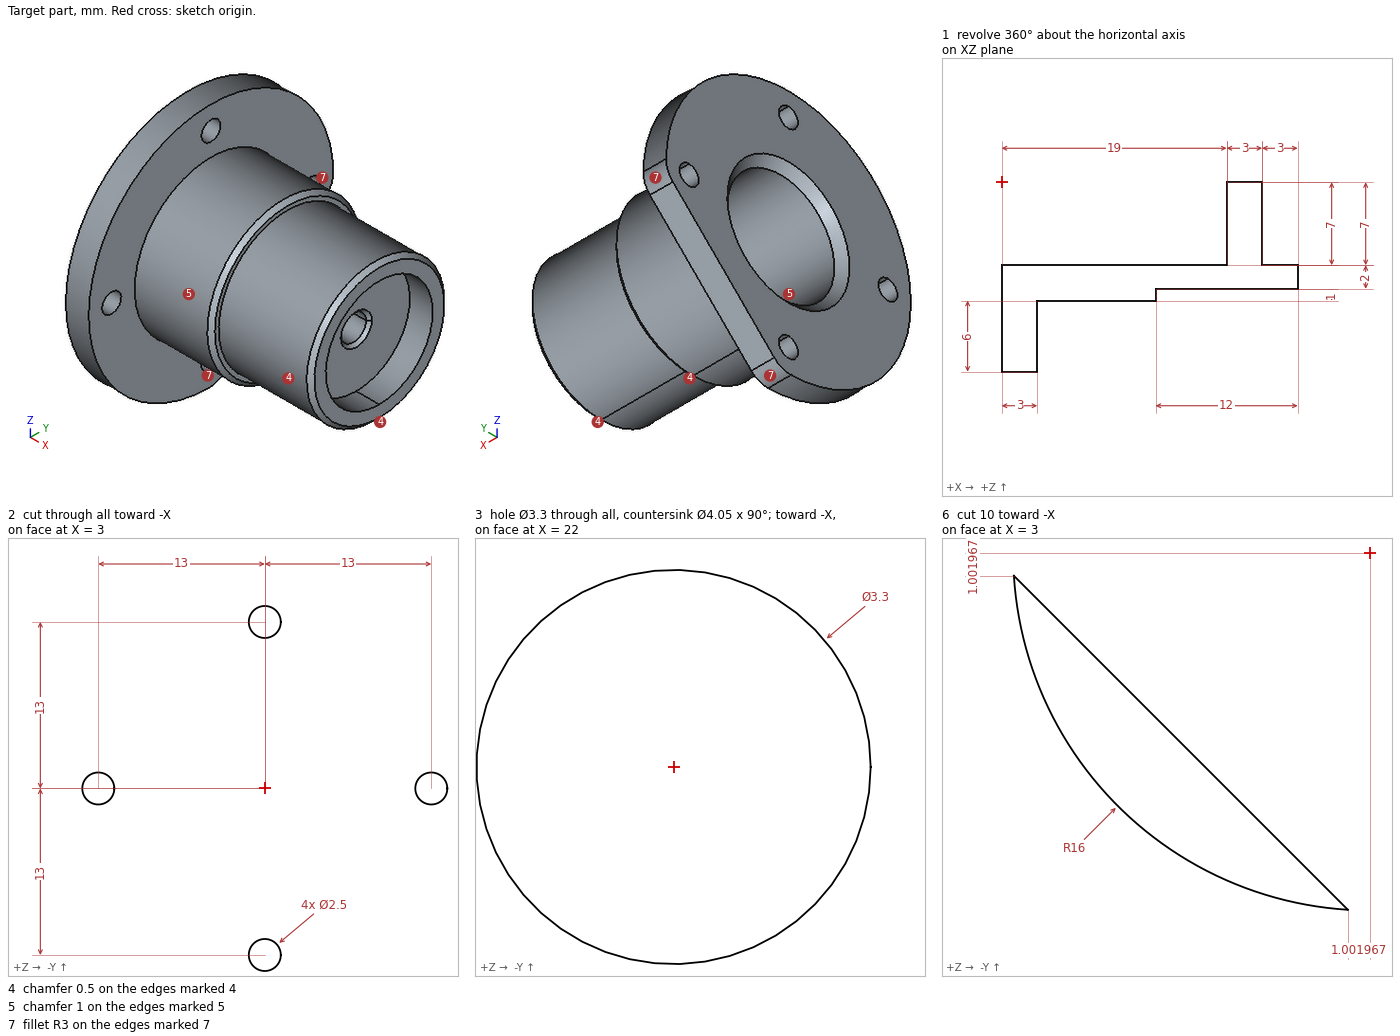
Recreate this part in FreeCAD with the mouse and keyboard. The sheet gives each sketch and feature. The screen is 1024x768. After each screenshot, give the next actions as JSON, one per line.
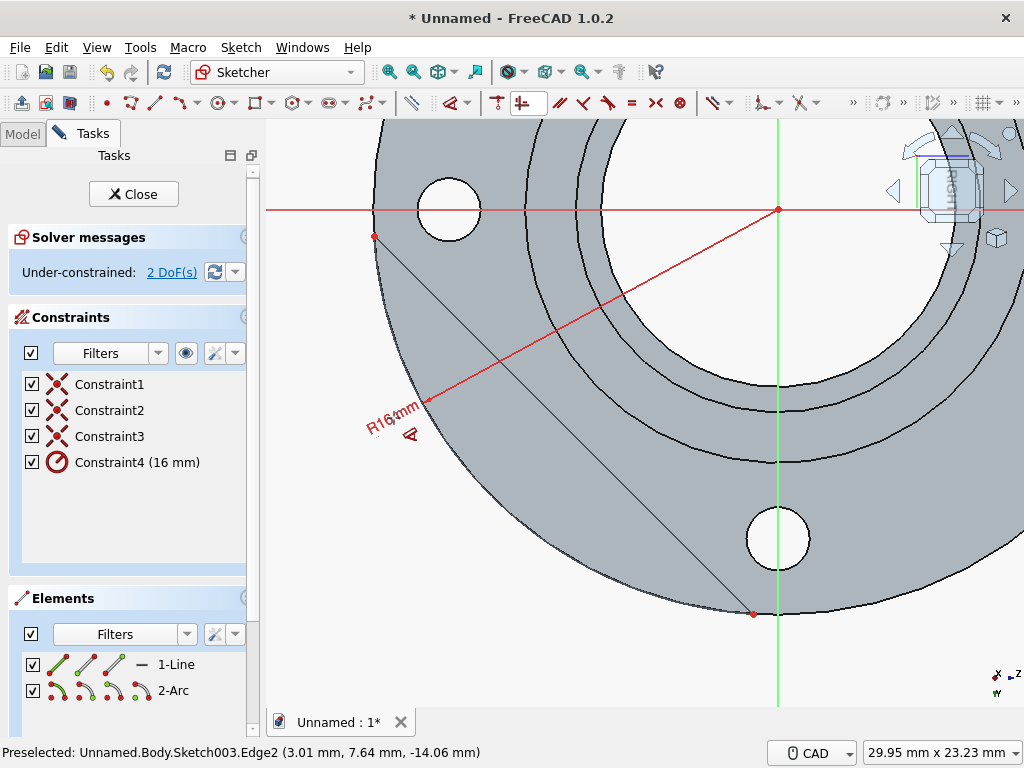
{"action": "scroll", "coordinate": [753, 614], "scroll_direction": "up", "scroll_amount": 3}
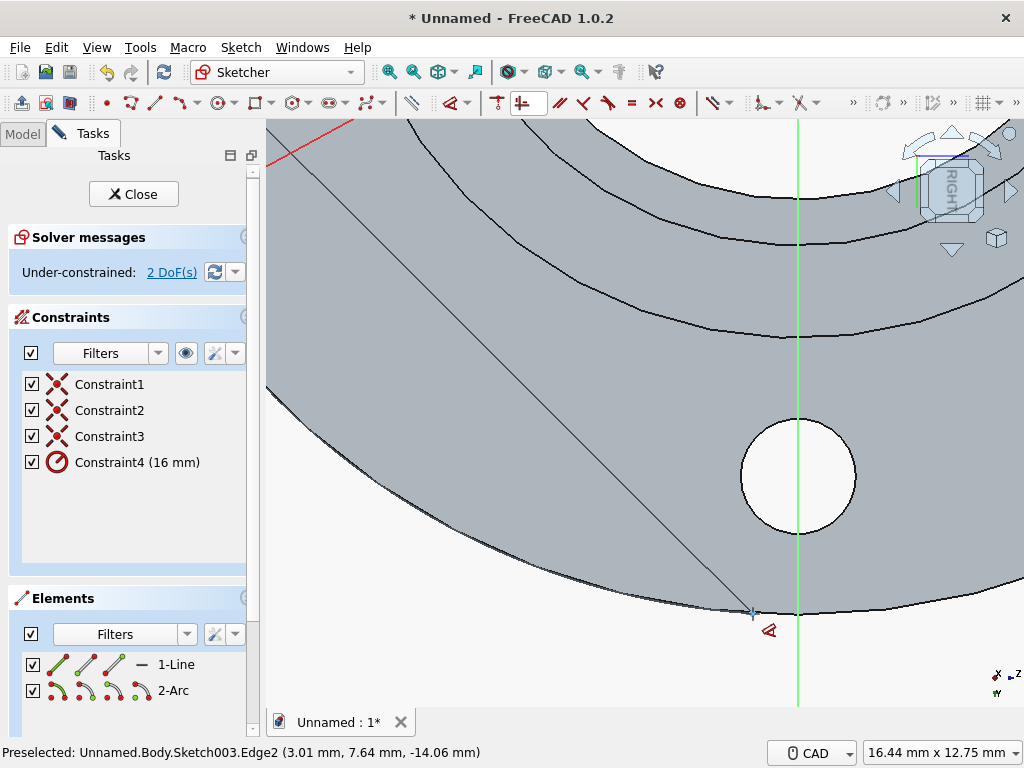
{"action": "left_click", "coordinate": [752, 613]}
{"action": "left_click", "coordinate": [775, 647]}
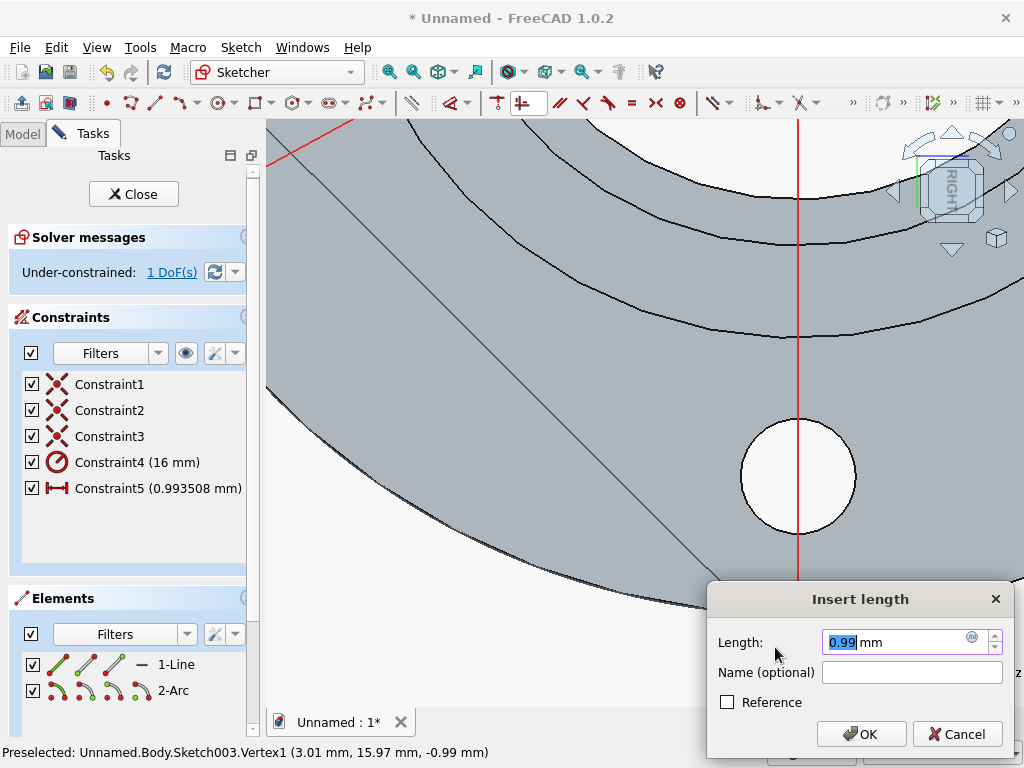
{"action": "type", "text": "1.001967"}
{"action": "key", "text": "Return"}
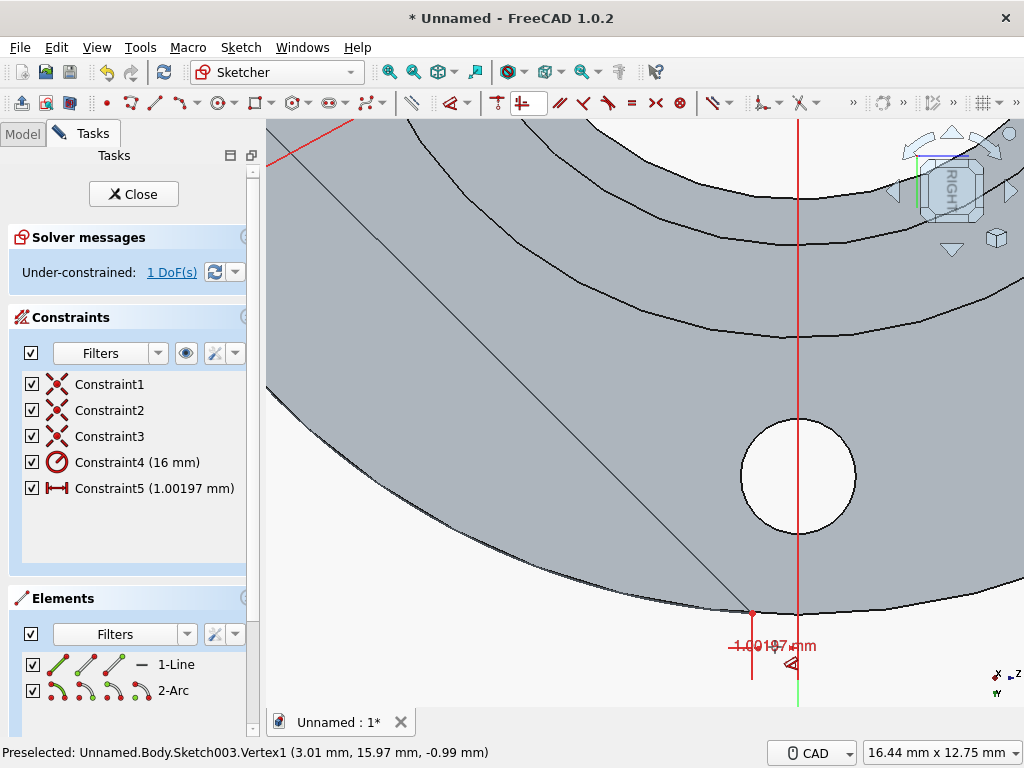
{"action": "scroll", "coordinate": [755, 617], "scroll_direction": "down", "scroll_amount": 3}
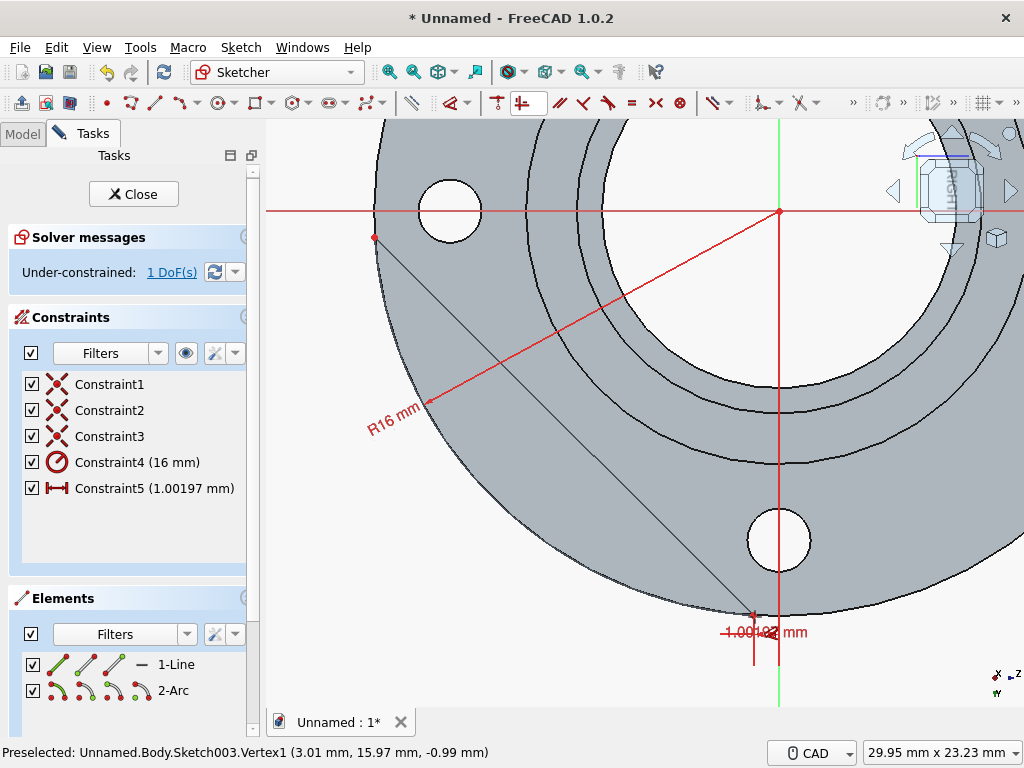
{"action": "scroll", "coordinate": [375, 237], "scroll_direction": "up", "scroll_amount": 3}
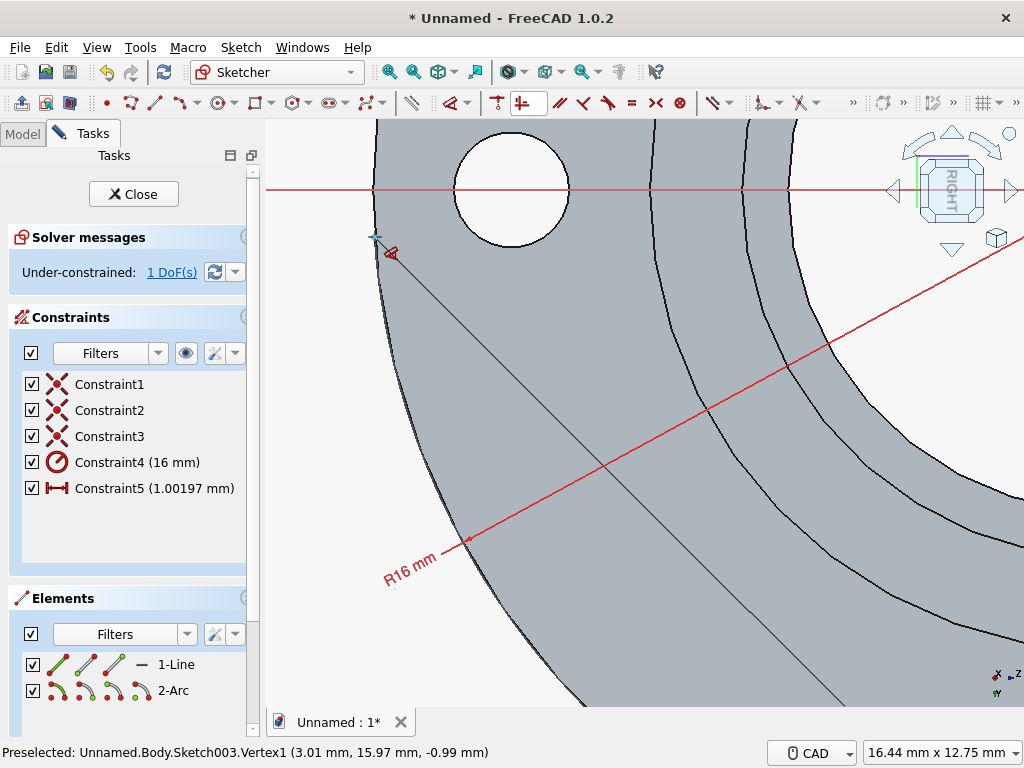
{"action": "left_click", "coordinate": [375, 237]}
{"action": "left_click", "coordinate": [341, 214]}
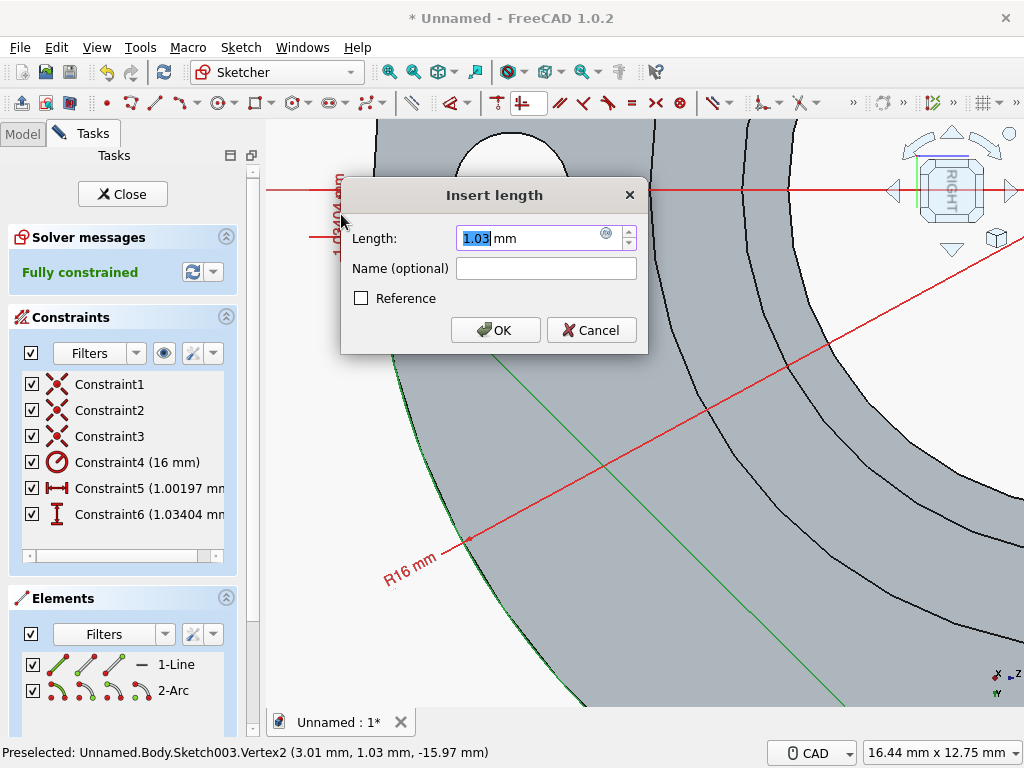
{"action": "type", "text": "1.001967"}
{"action": "key", "text": "Return"}
{"action": "key", "text": "Escape"}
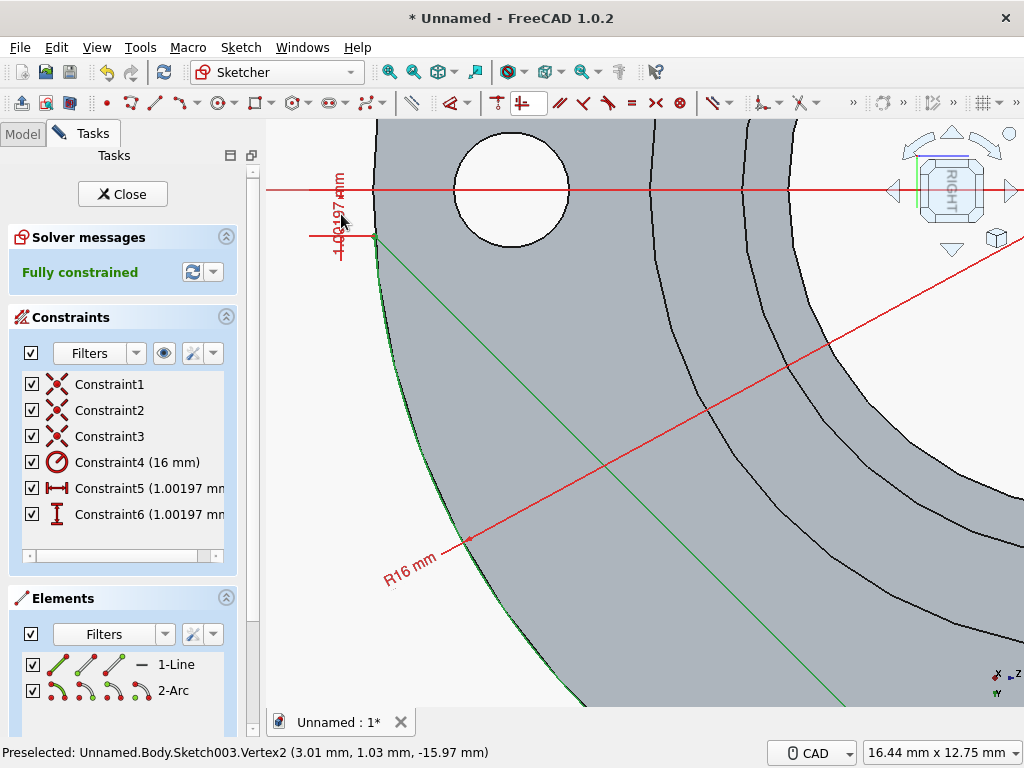
{"action": "left_click", "coordinate": [123, 194]}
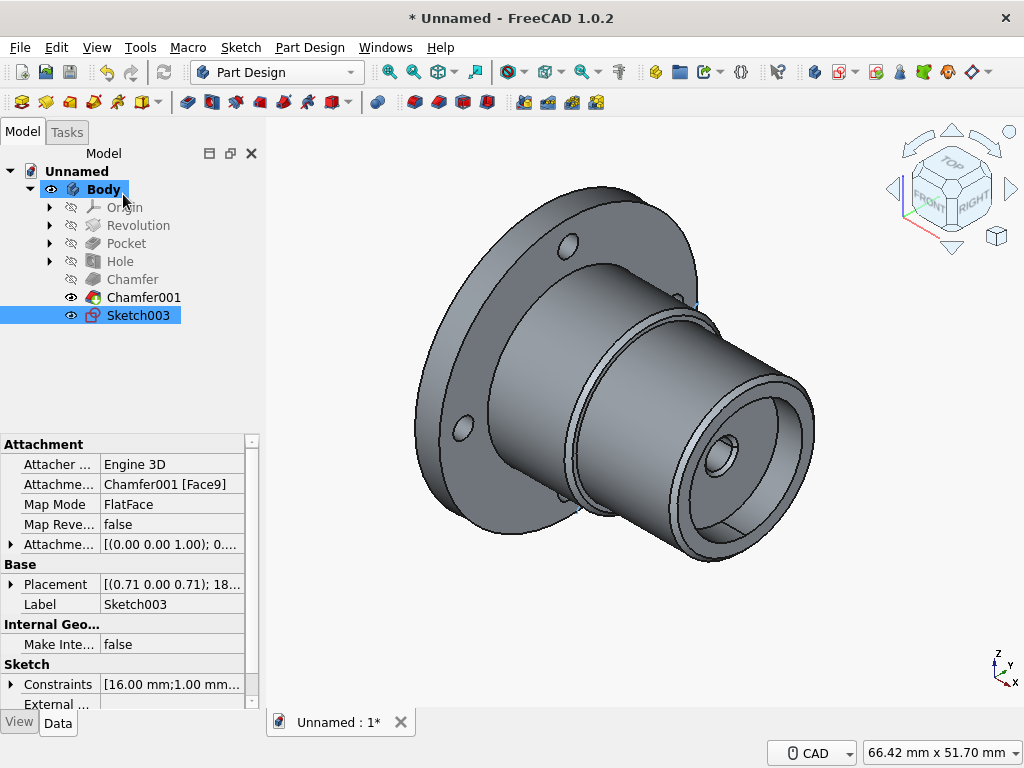
{"action": "left_click", "coordinate": [188, 102]}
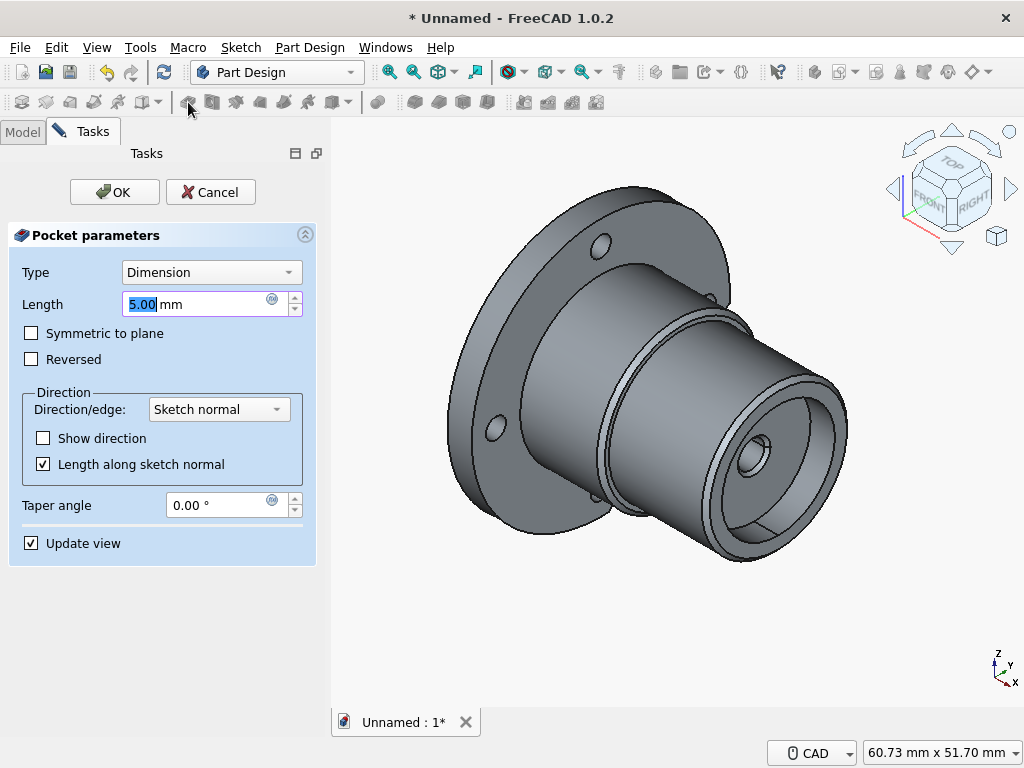
{"action": "type", "text": "10"}
{"action": "key", "text": "Tab"}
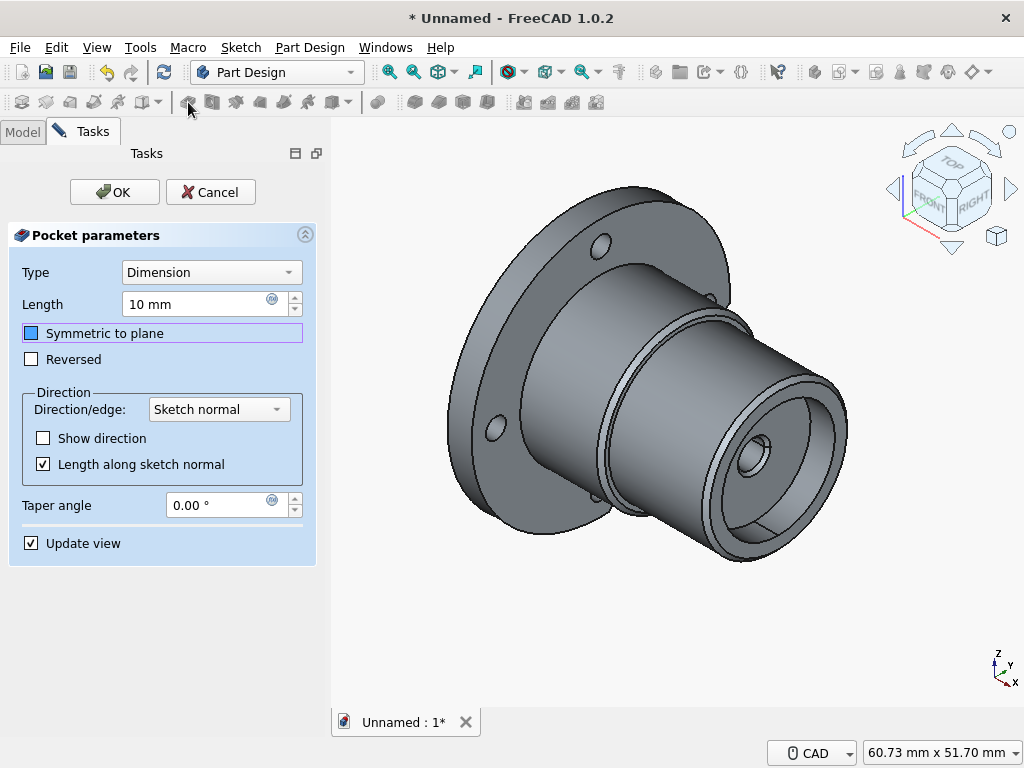
{"action": "left_click", "coordinate": [115, 192]}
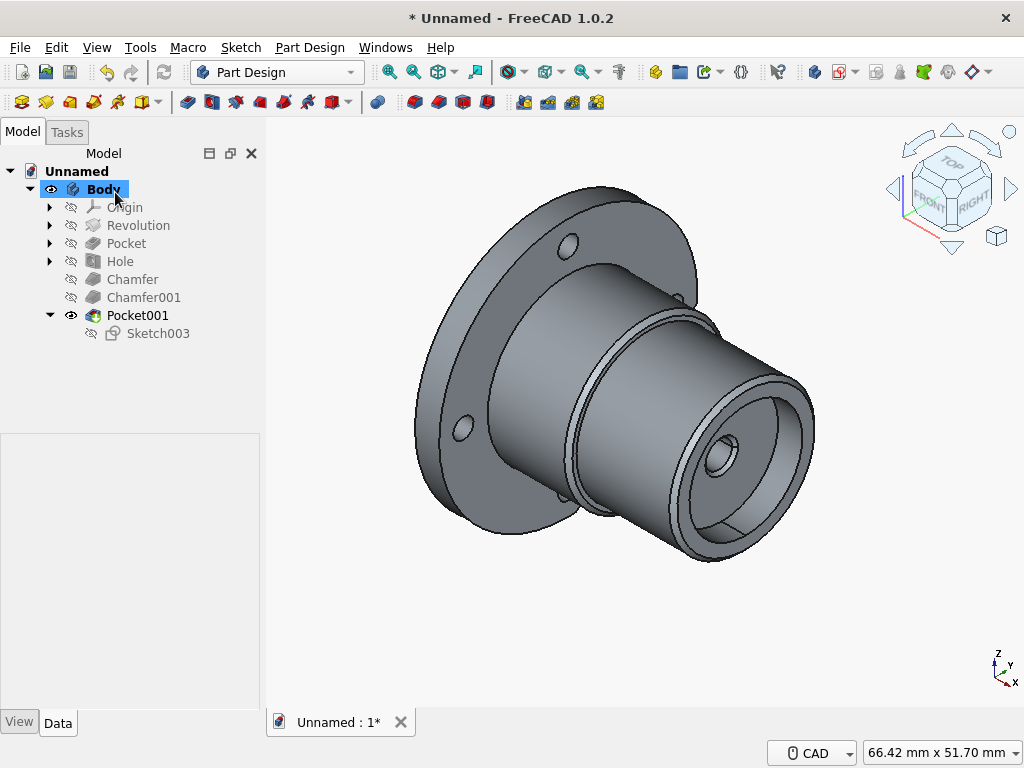
{"action": "key", "text": "2"}